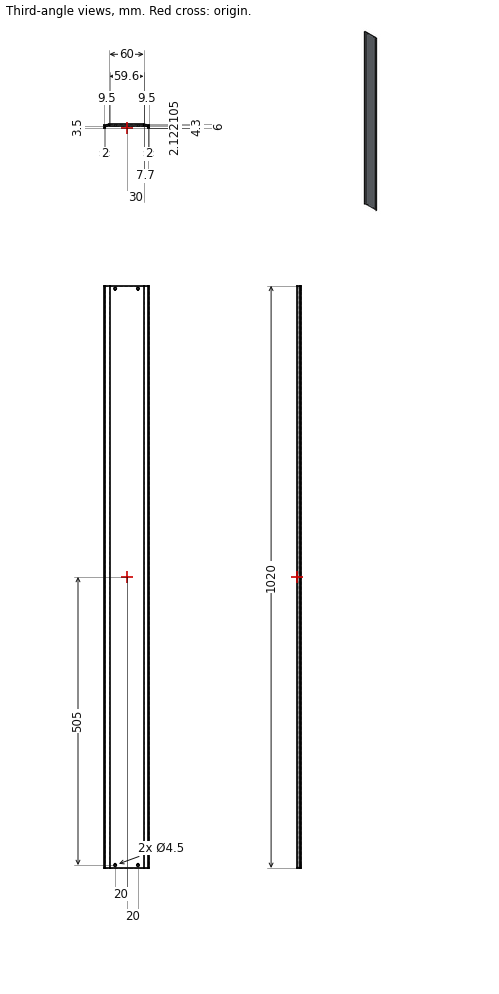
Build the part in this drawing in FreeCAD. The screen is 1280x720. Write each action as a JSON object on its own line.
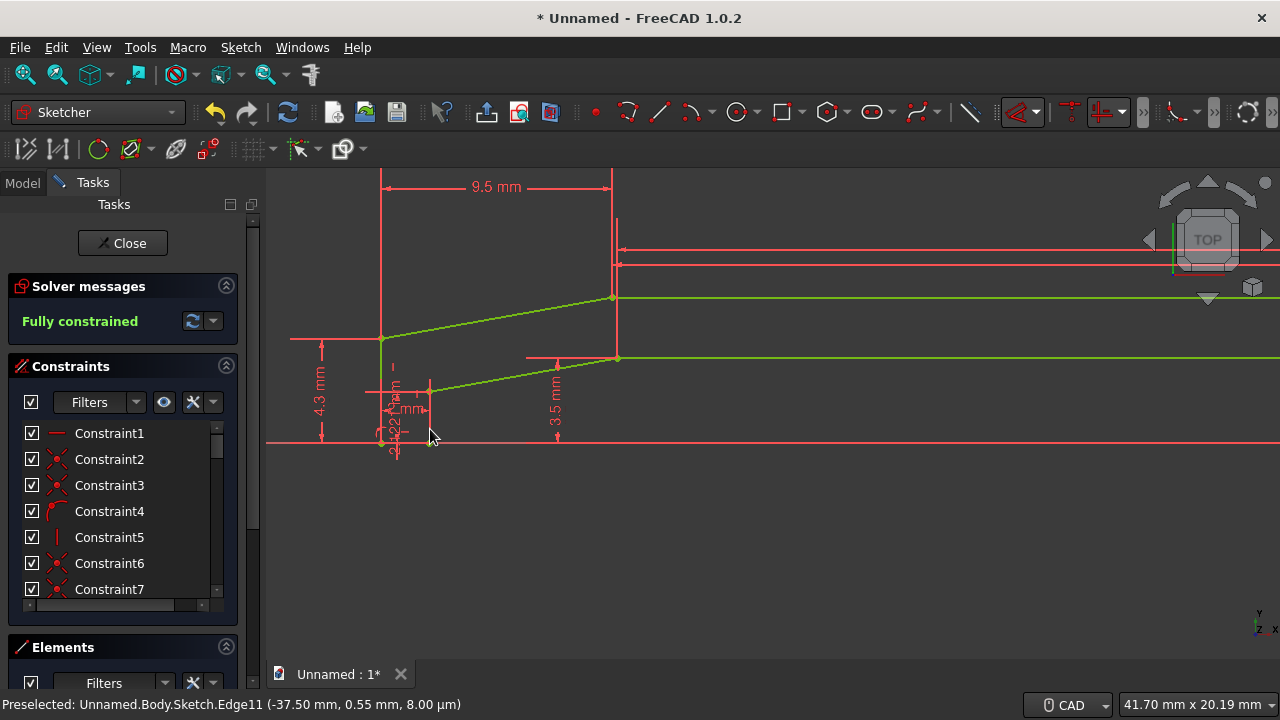
{"action": "left_click", "coordinate": [123, 243]}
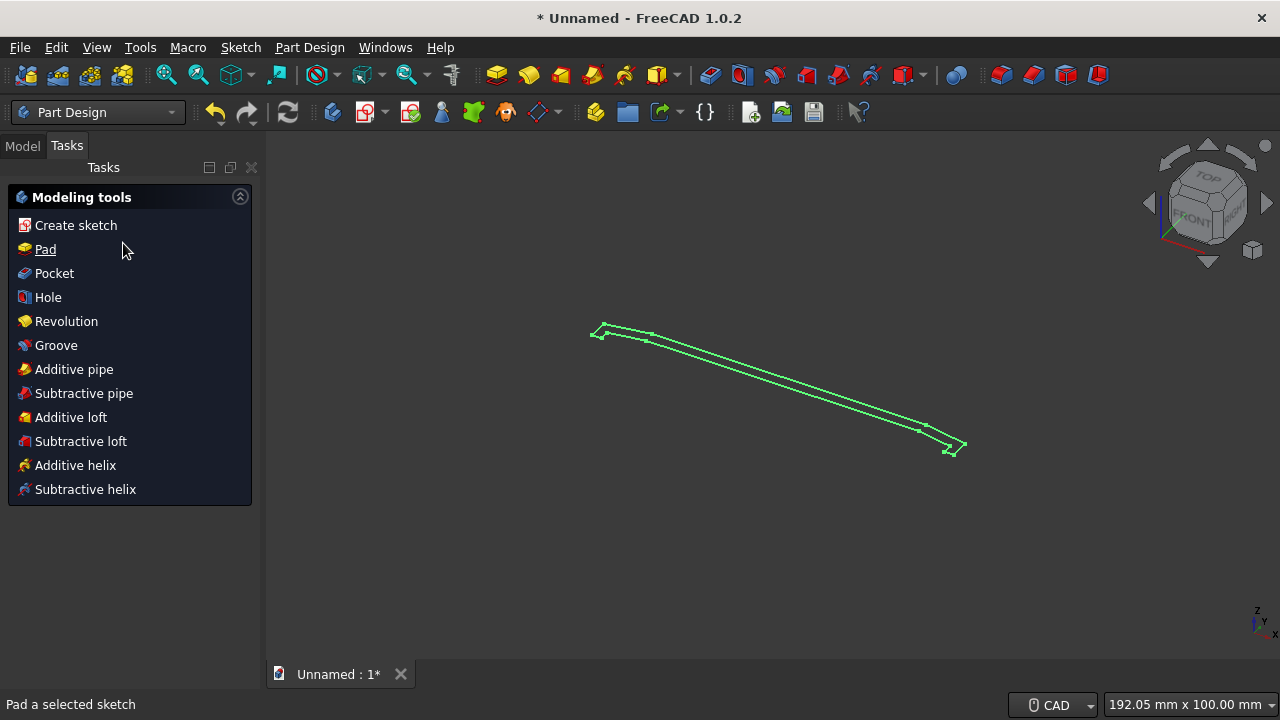
{"action": "left_click", "coordinate": [498, 76]}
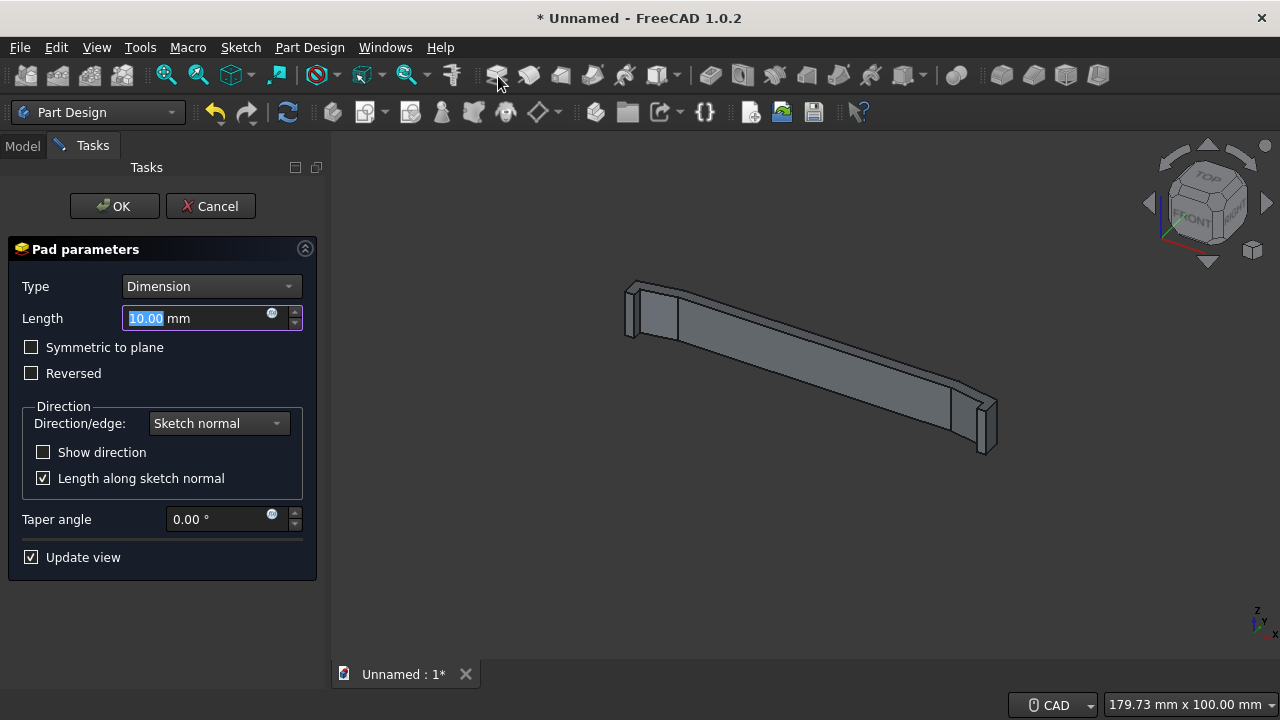
{"action": "type", "text": "1020"}
{"action": "key", "text": "Tab"}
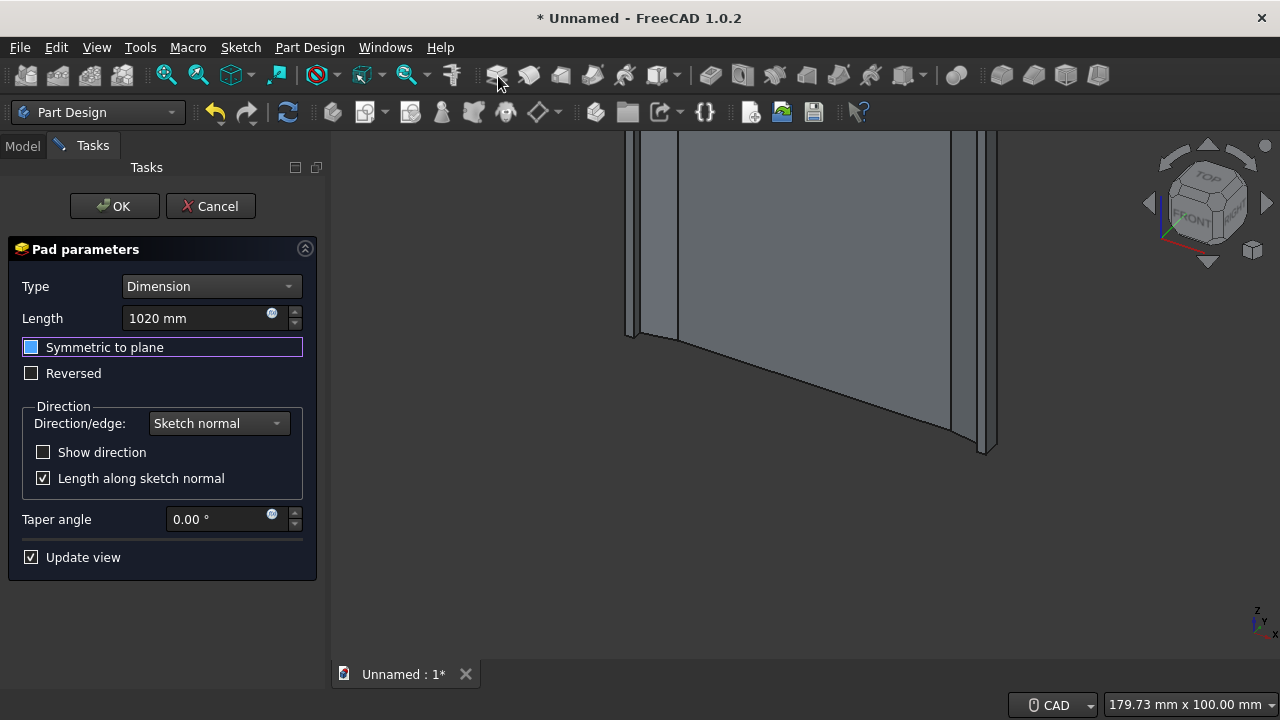
{"action": "left_click", "coordinate": [30, 347]}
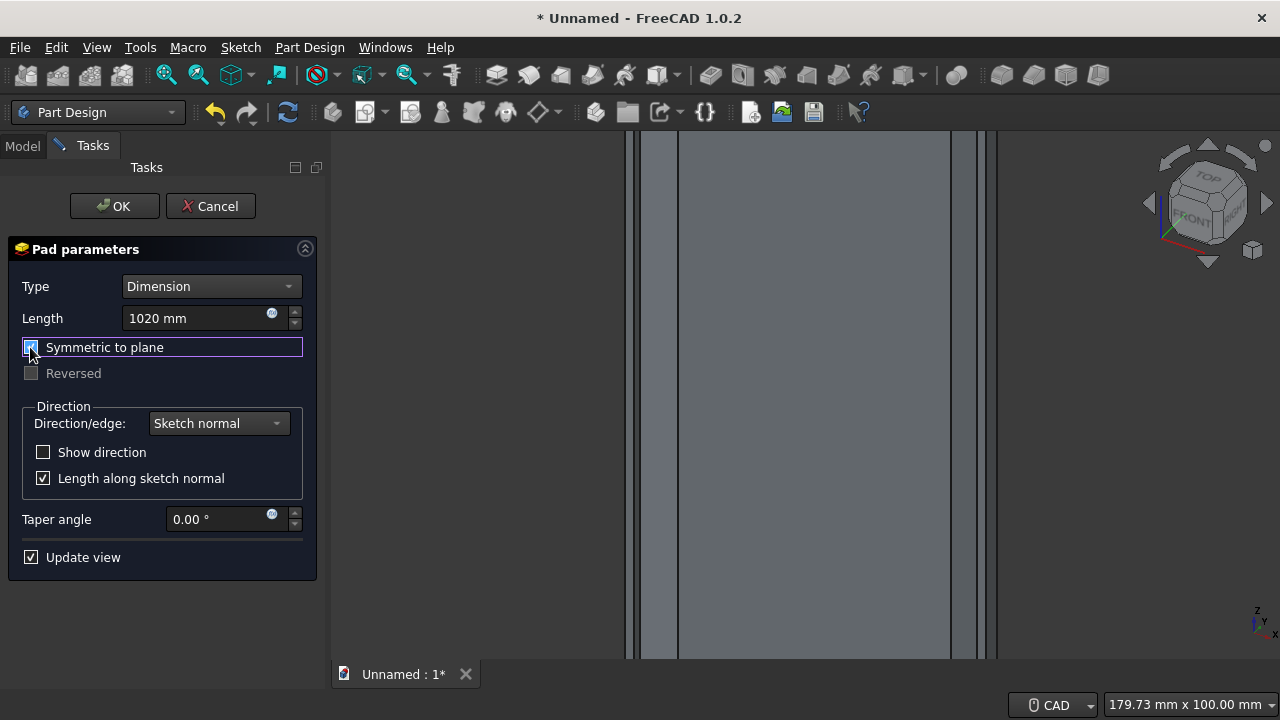
{"action": "left_click", "coordinate": [115, 206]}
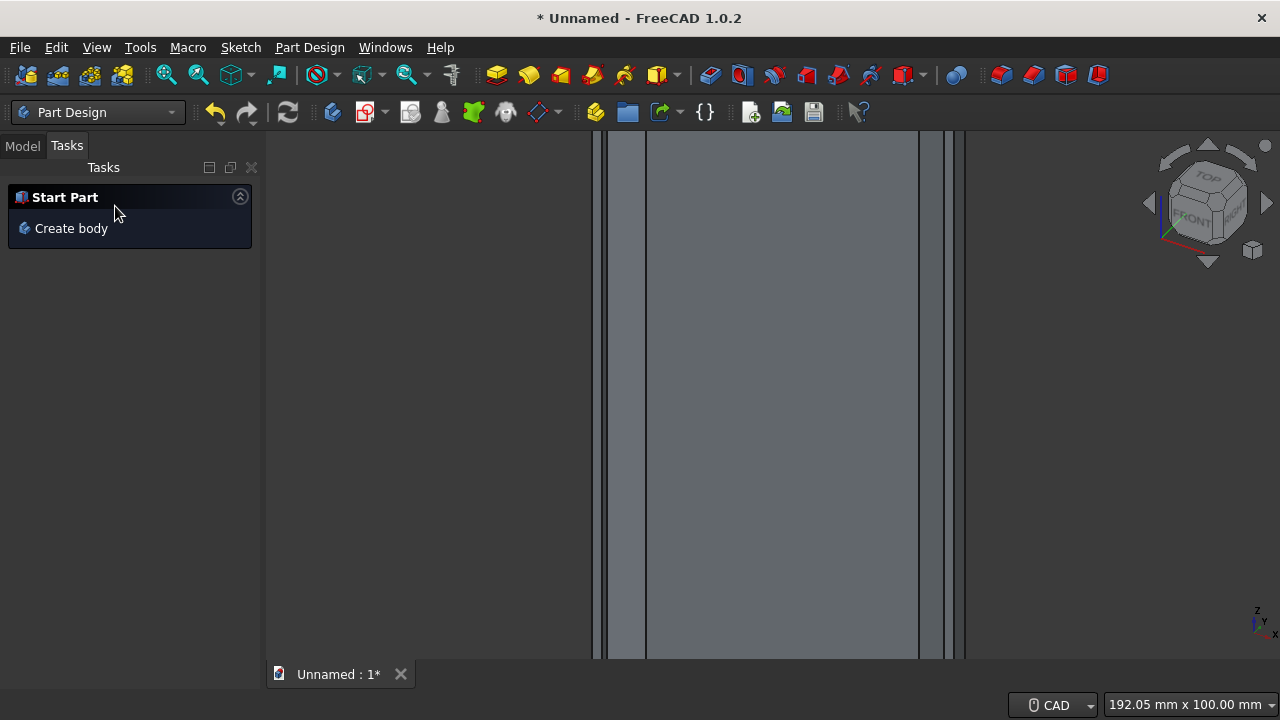
{"action": "key", "text": "v f"}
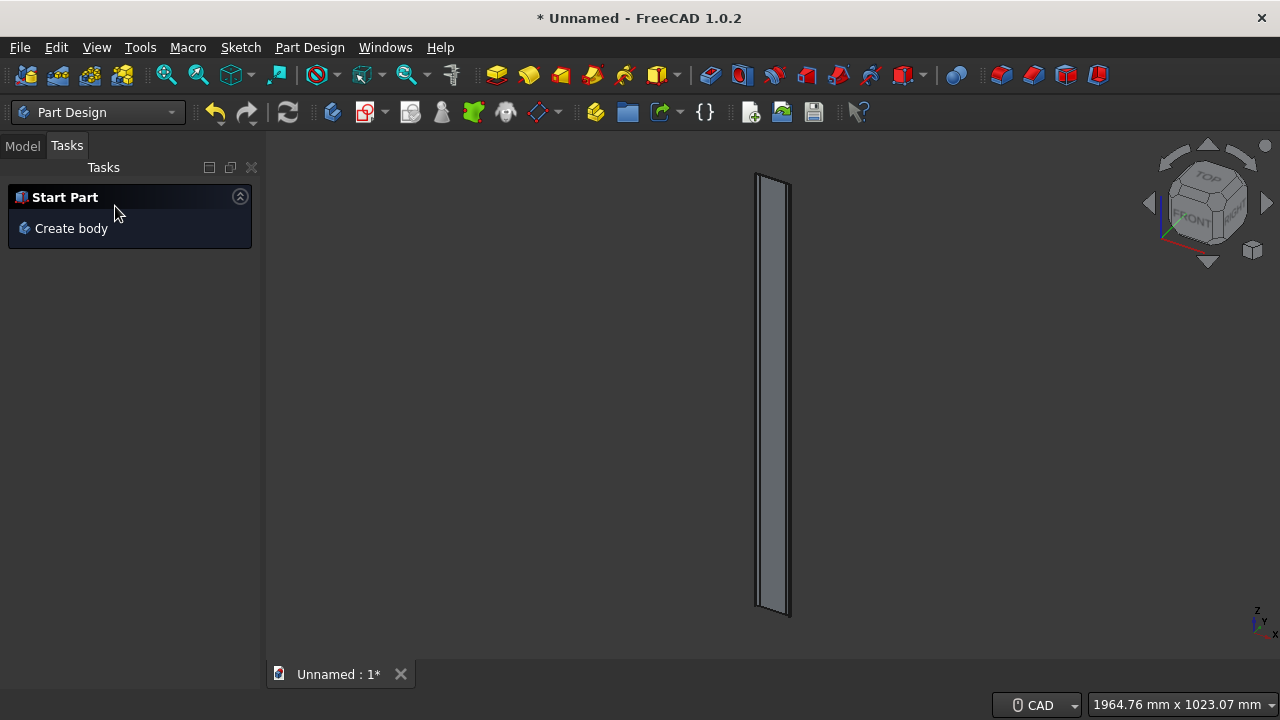
{"action": "key", "text": "4"}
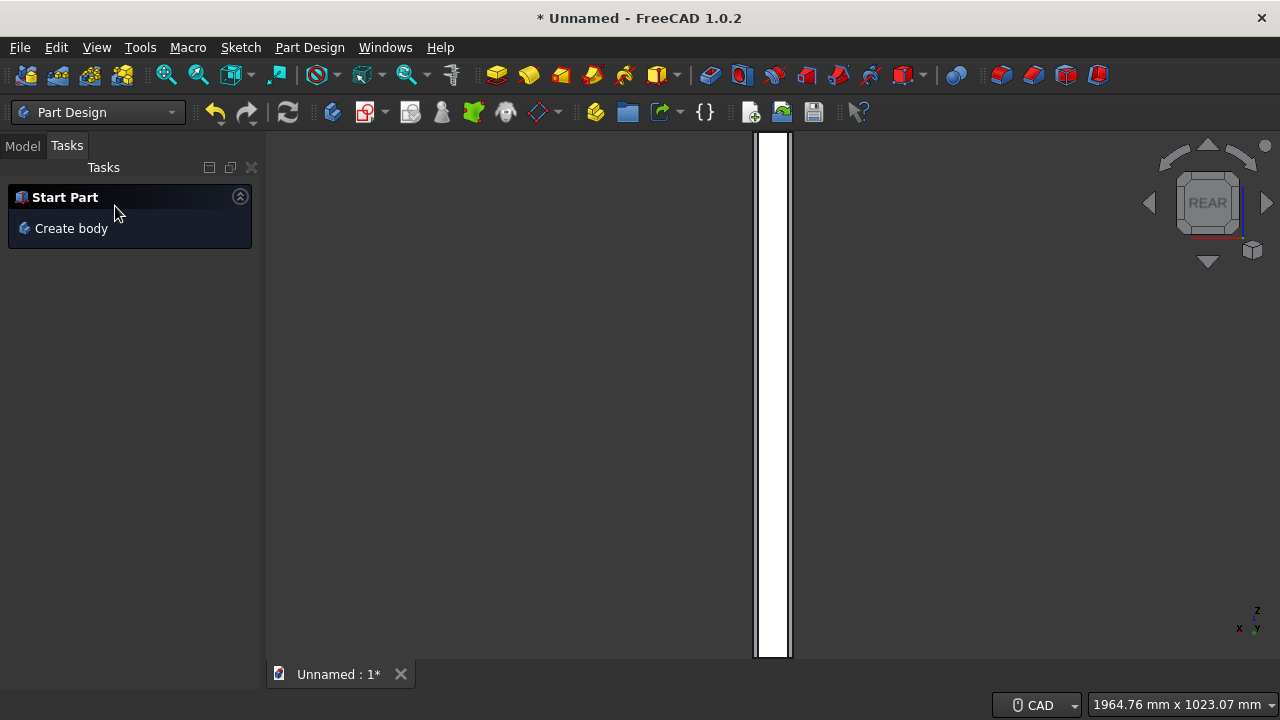
{"action": "left_click", "coordinate": [773, 168]}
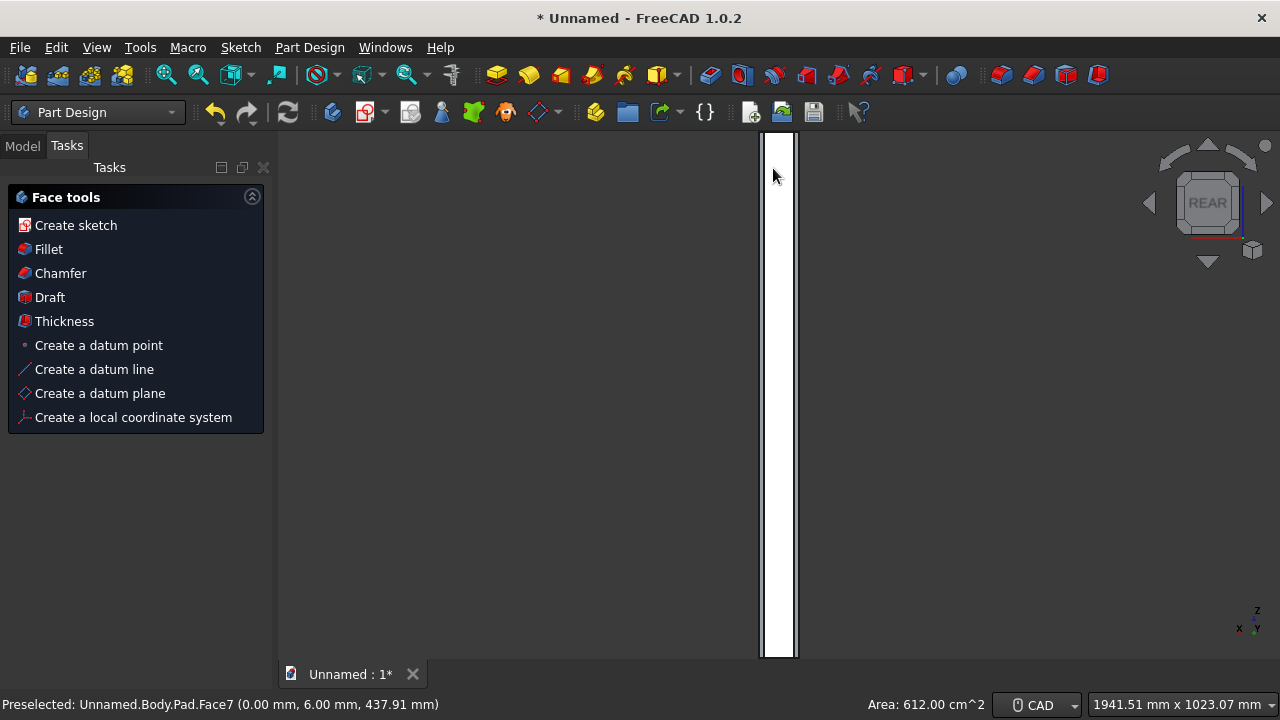
{"action": "left_click", "coordinate": [366, 112]}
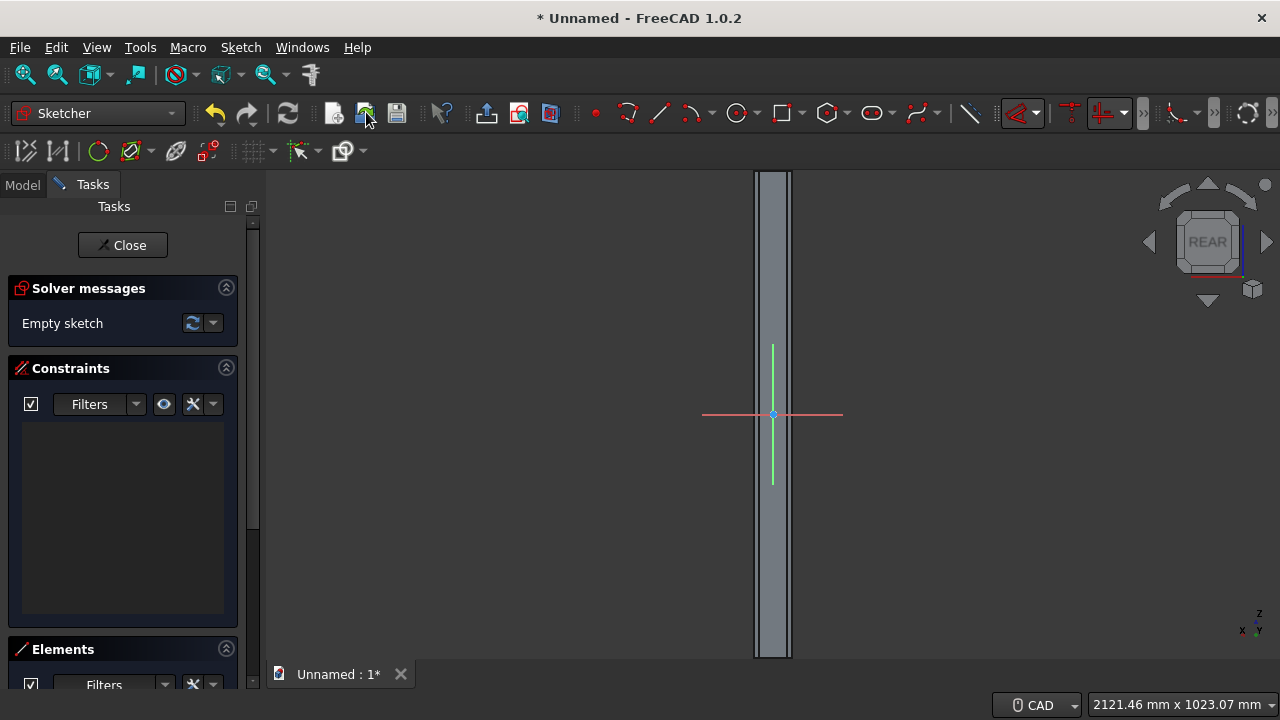
{"action": "scroll", "coordinate": [704, 414], "scroll_direction": "down", "scroll_amount": 5}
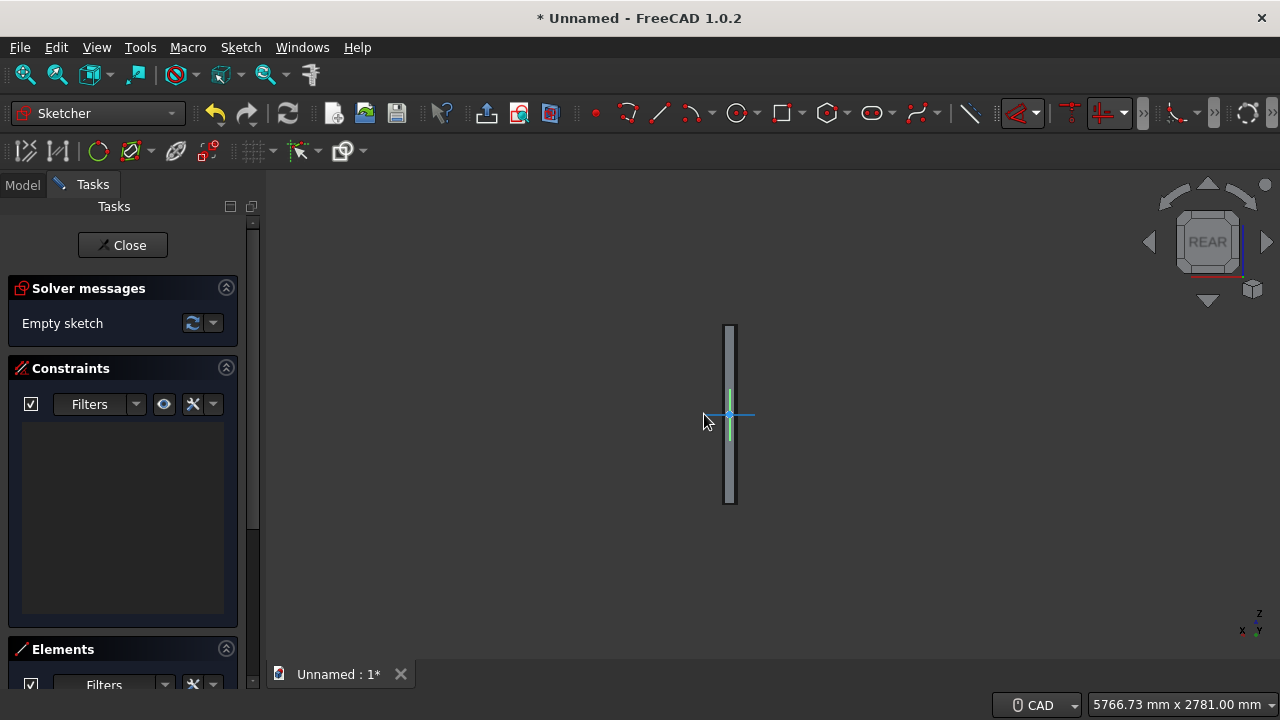
{"action": "scroll", "coordinate": [731, 508], "scroll_direction": "up", "scroll_amount": 15}